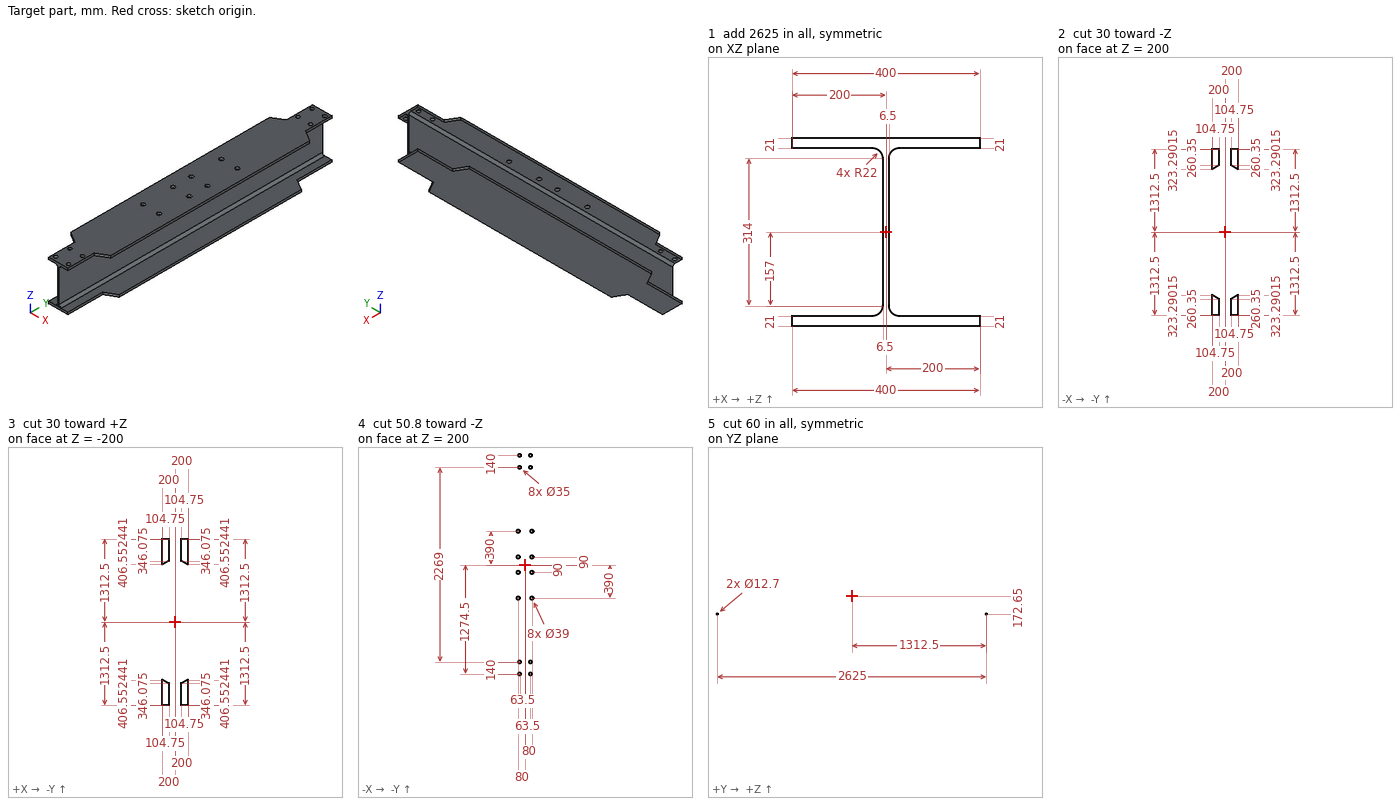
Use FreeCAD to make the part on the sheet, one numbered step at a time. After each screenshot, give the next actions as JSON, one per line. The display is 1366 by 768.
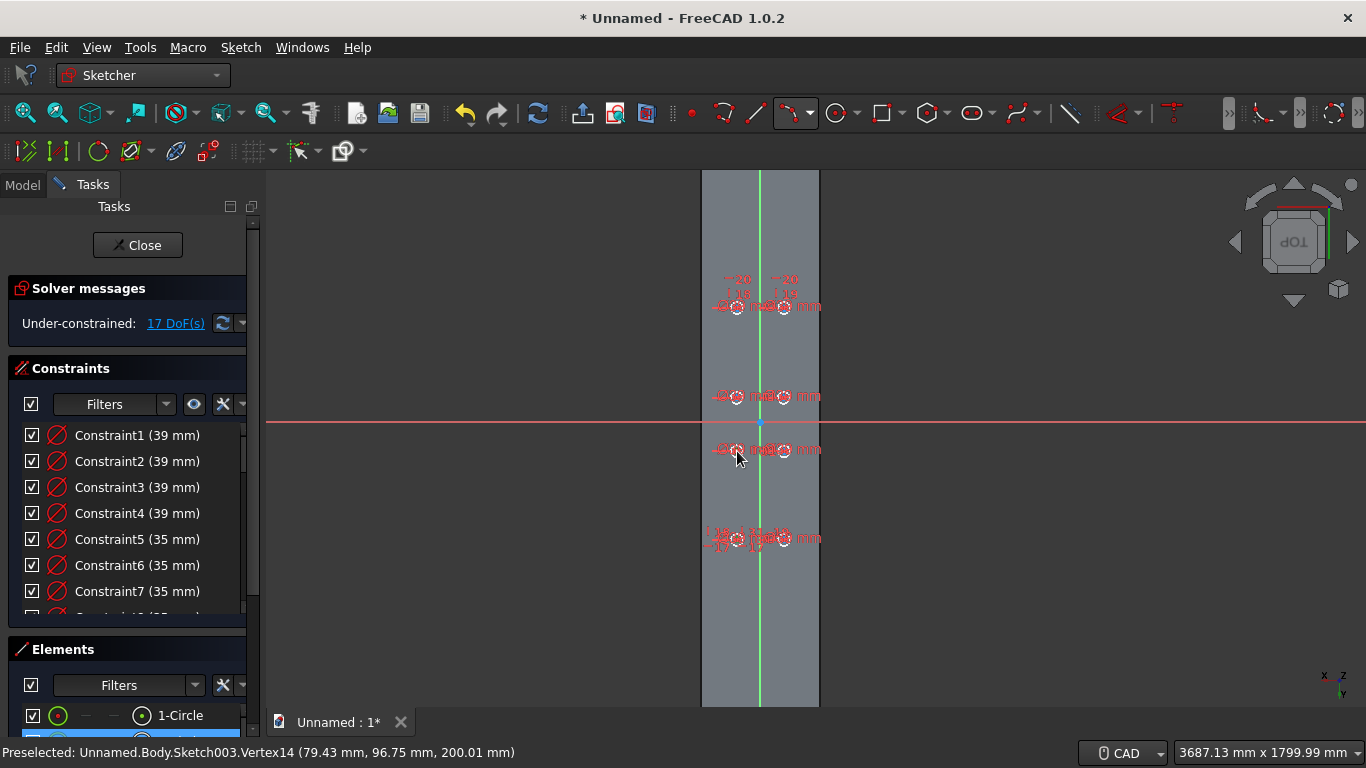
{"action": "key", "text": "v"}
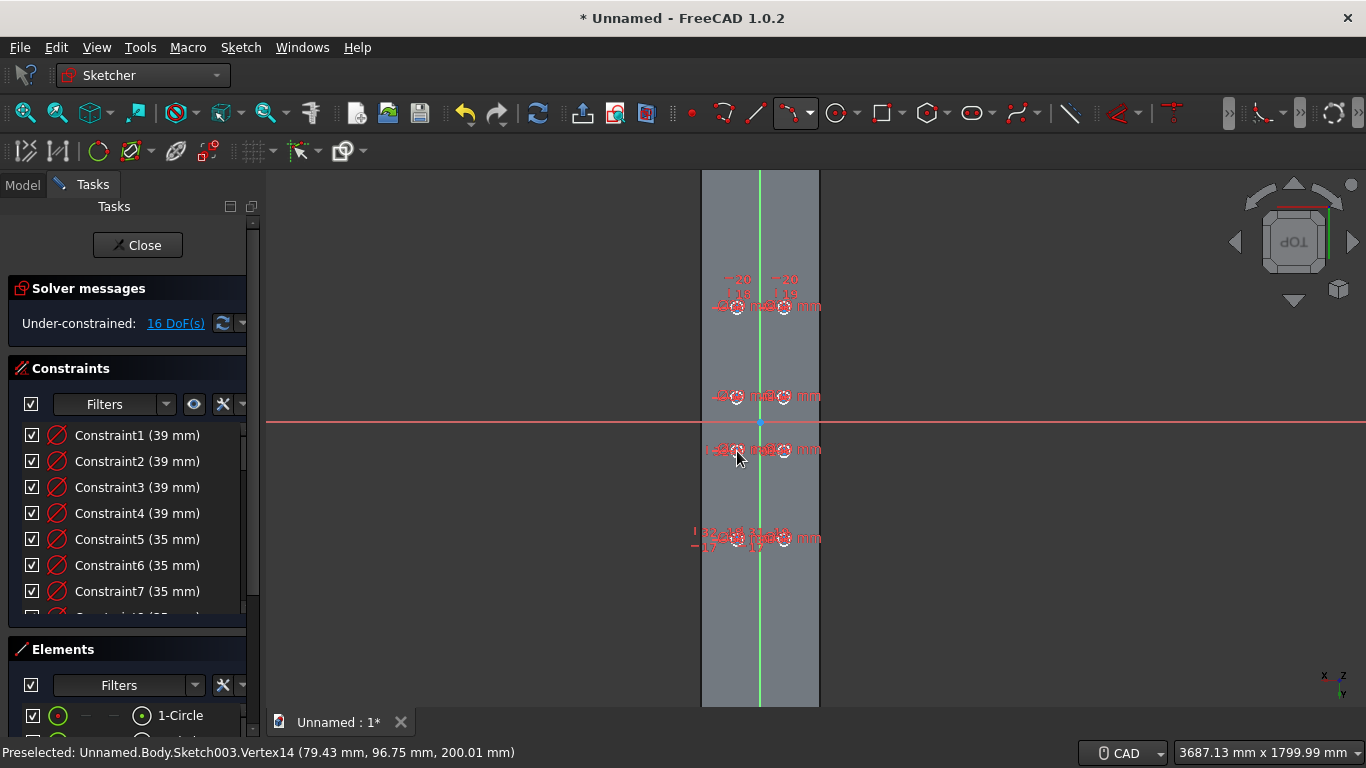
{"action": "left_click", "coordinate": [784, 451]}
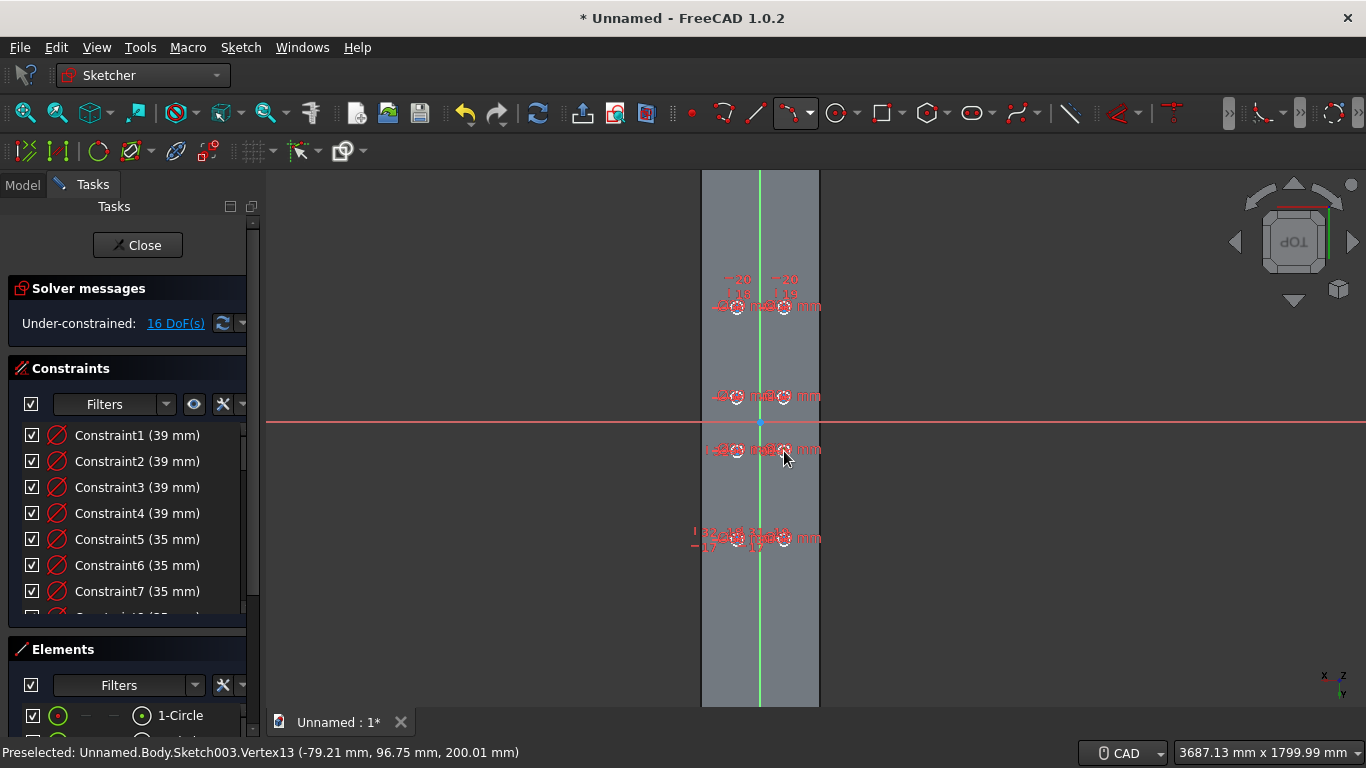
{"action": "left_click", "coordinate": [737, 451]}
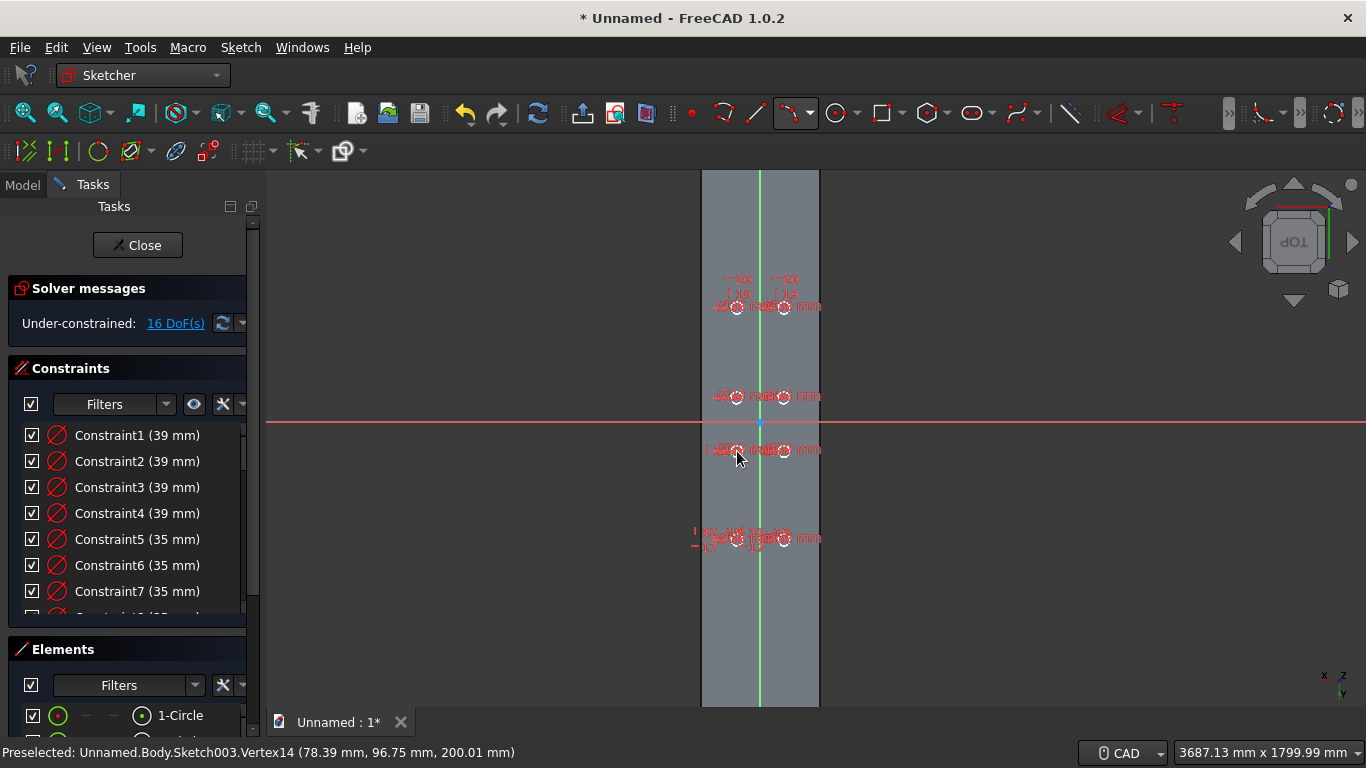
{"action": "key", "text": "h"}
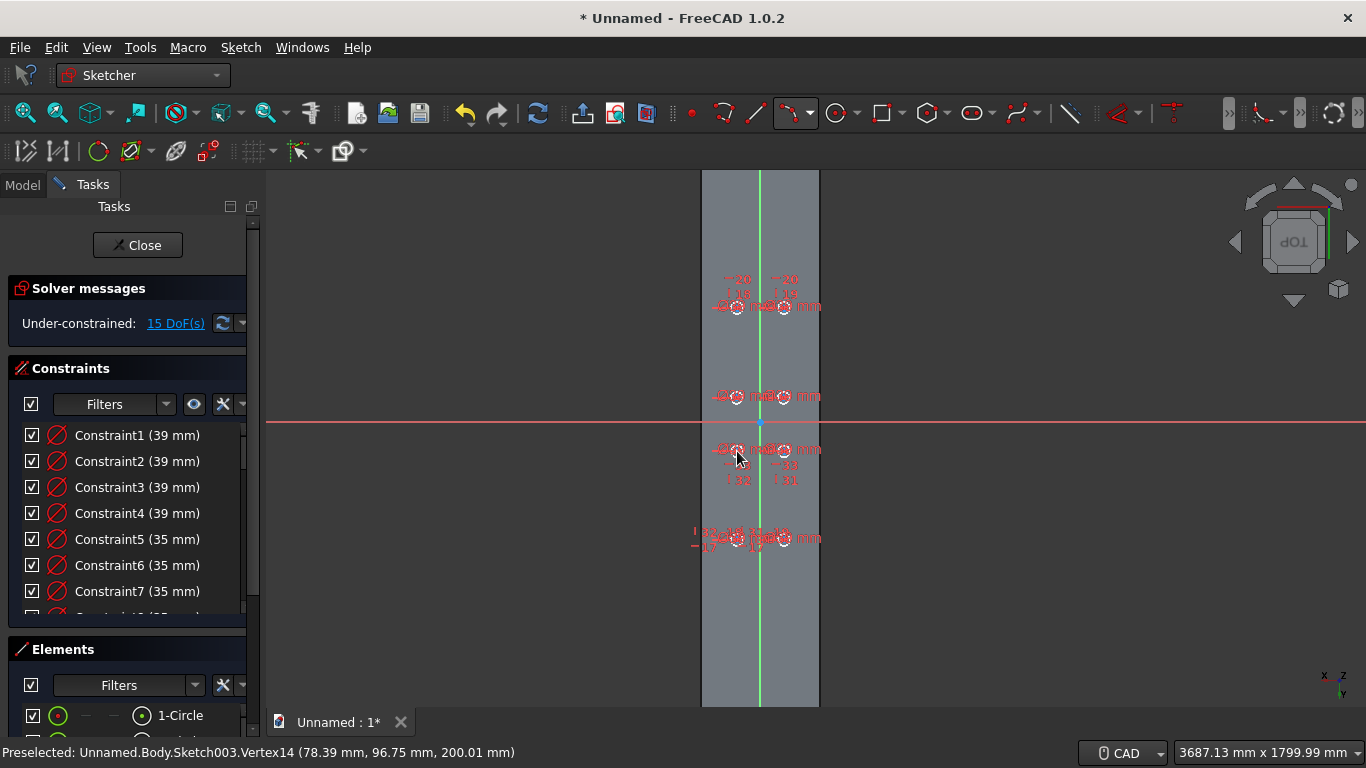
{"action": "left_click", "coordinate": [784, 451]}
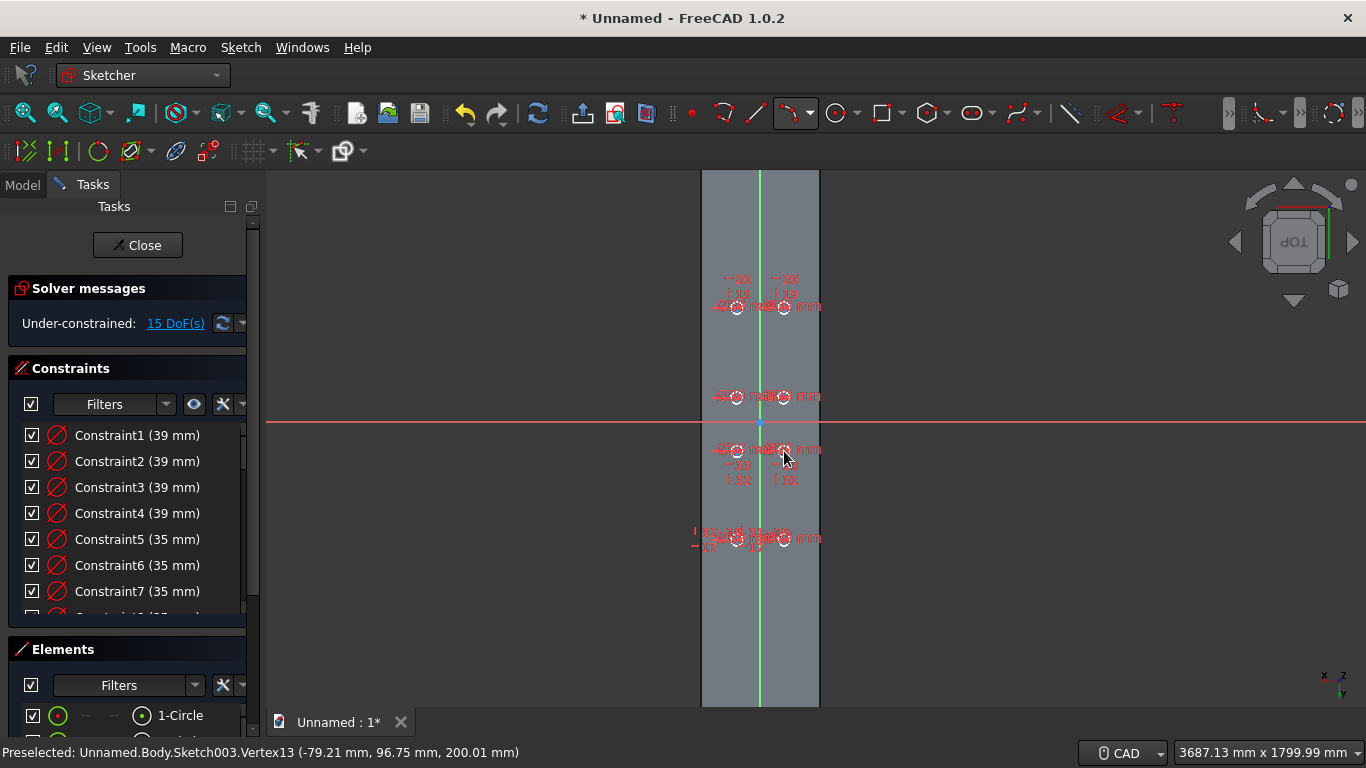
{"action": "left_click", "coordinate": [784, 398]}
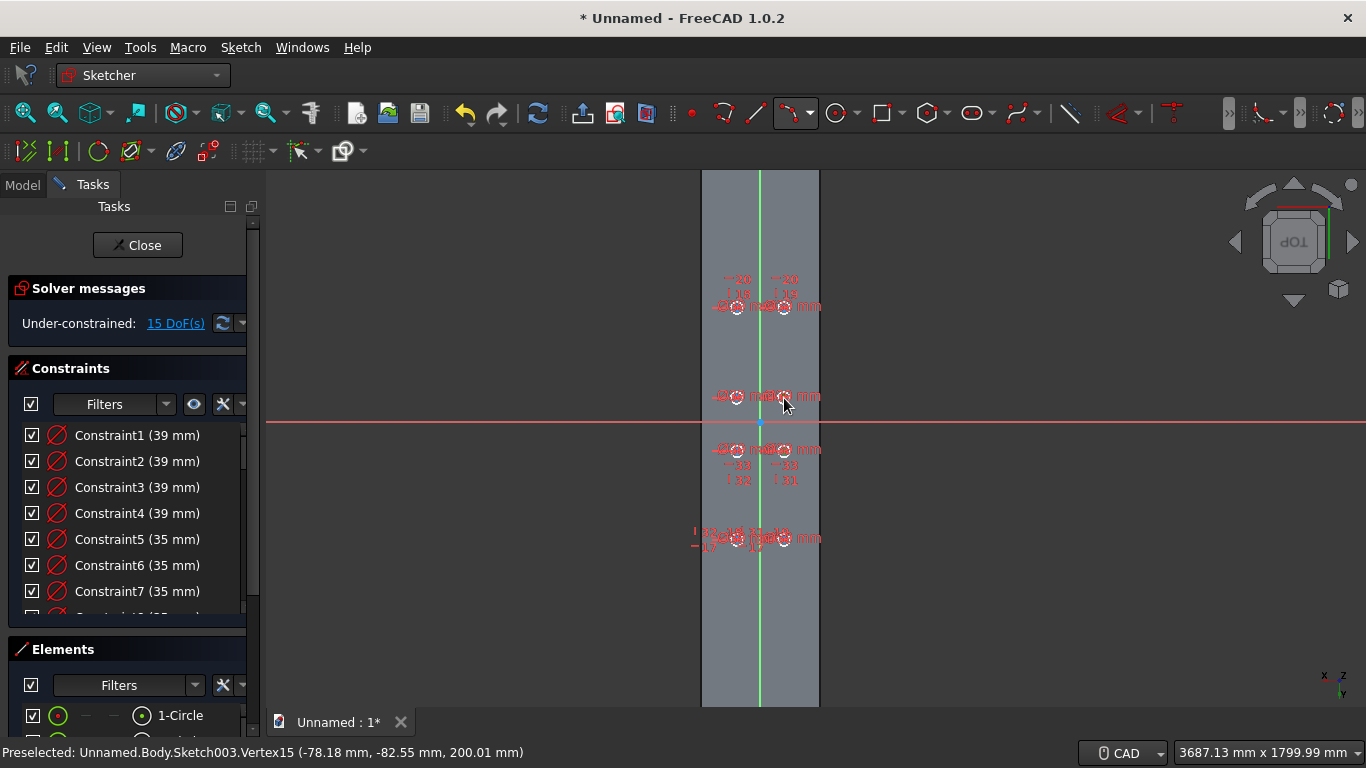
{"action": "key", "text": "v"}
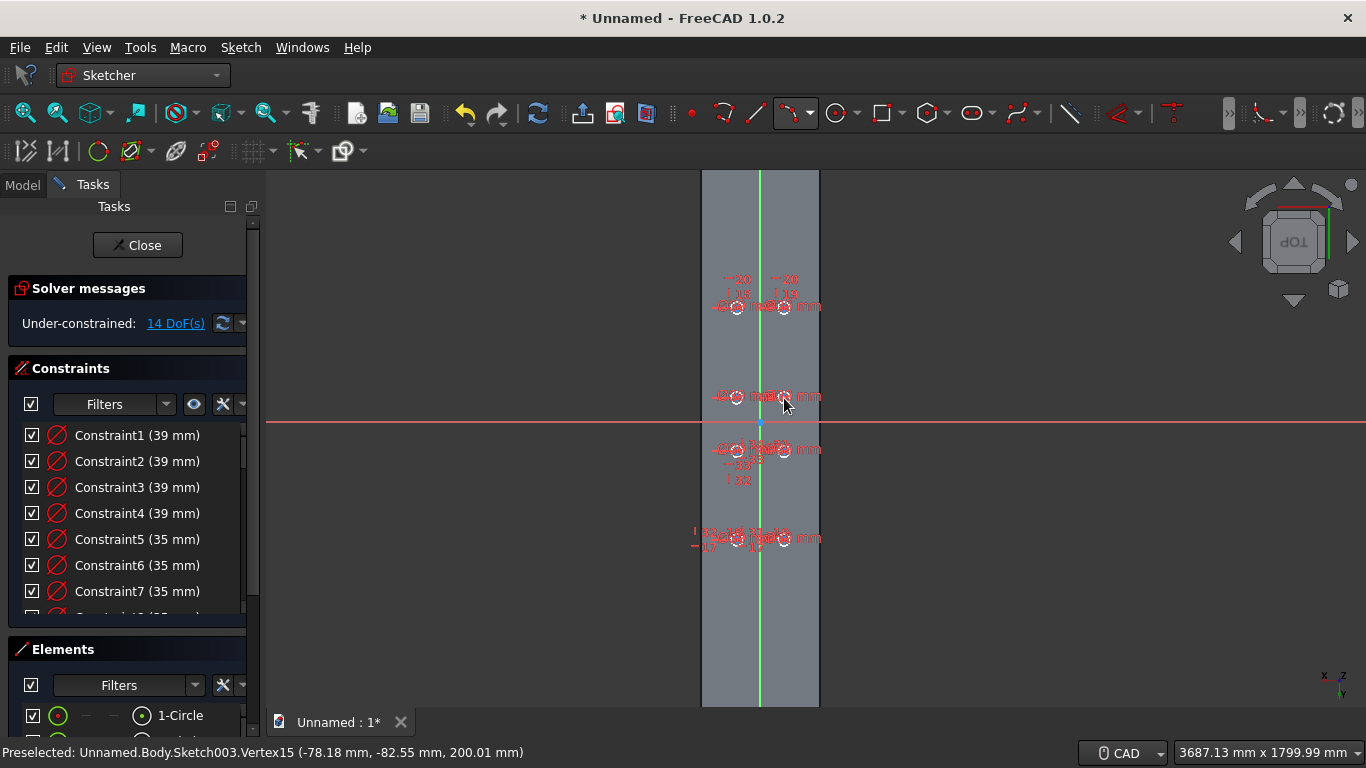
{"action": "left_click", "coordinate": [737, 451]}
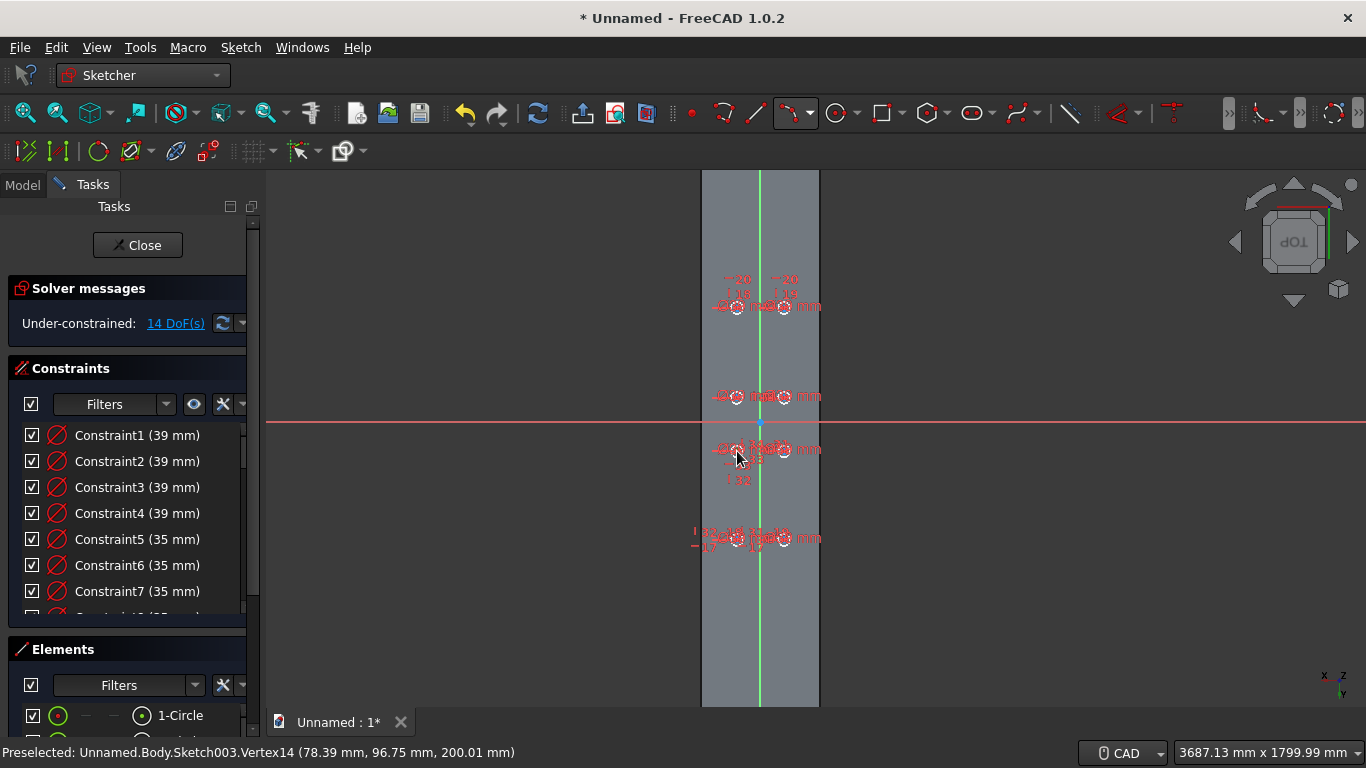
{"action": "left_click", "coordinate": [737, 398]}